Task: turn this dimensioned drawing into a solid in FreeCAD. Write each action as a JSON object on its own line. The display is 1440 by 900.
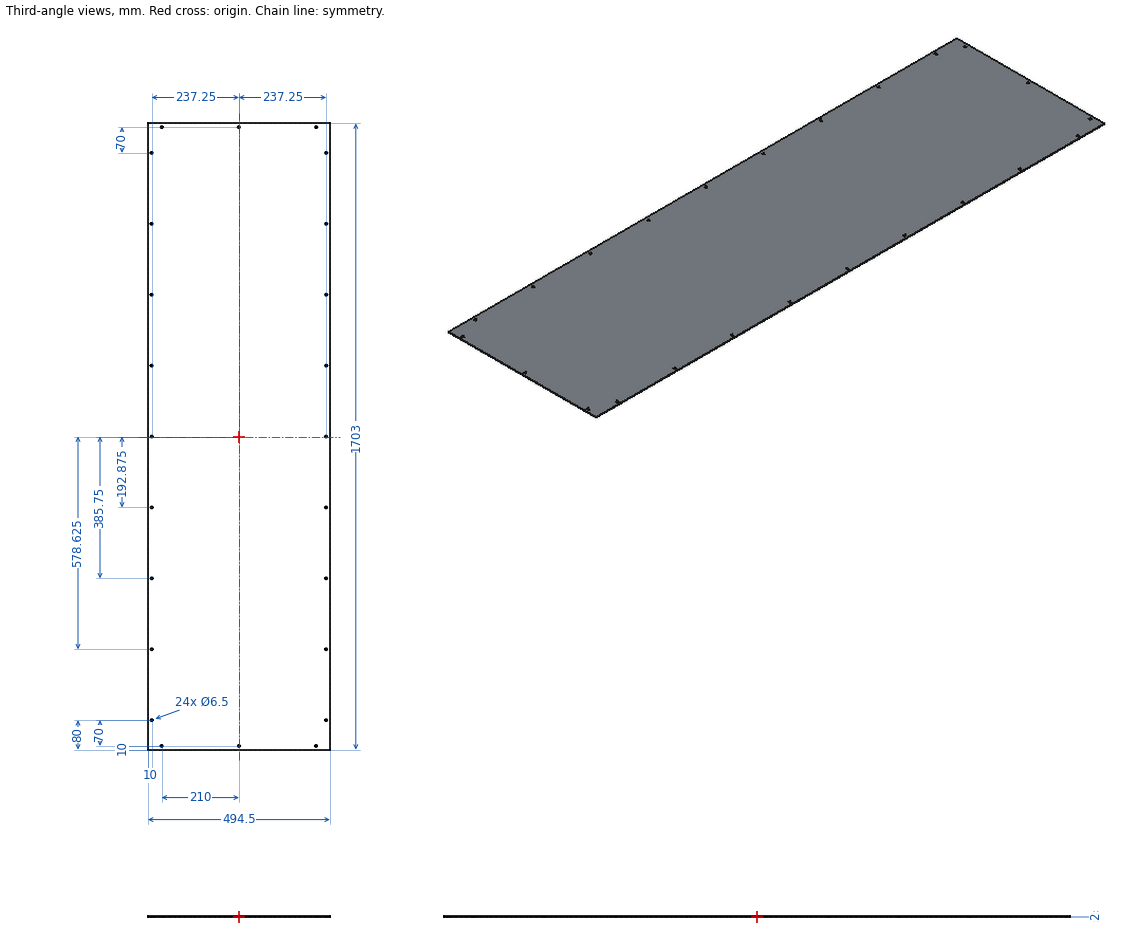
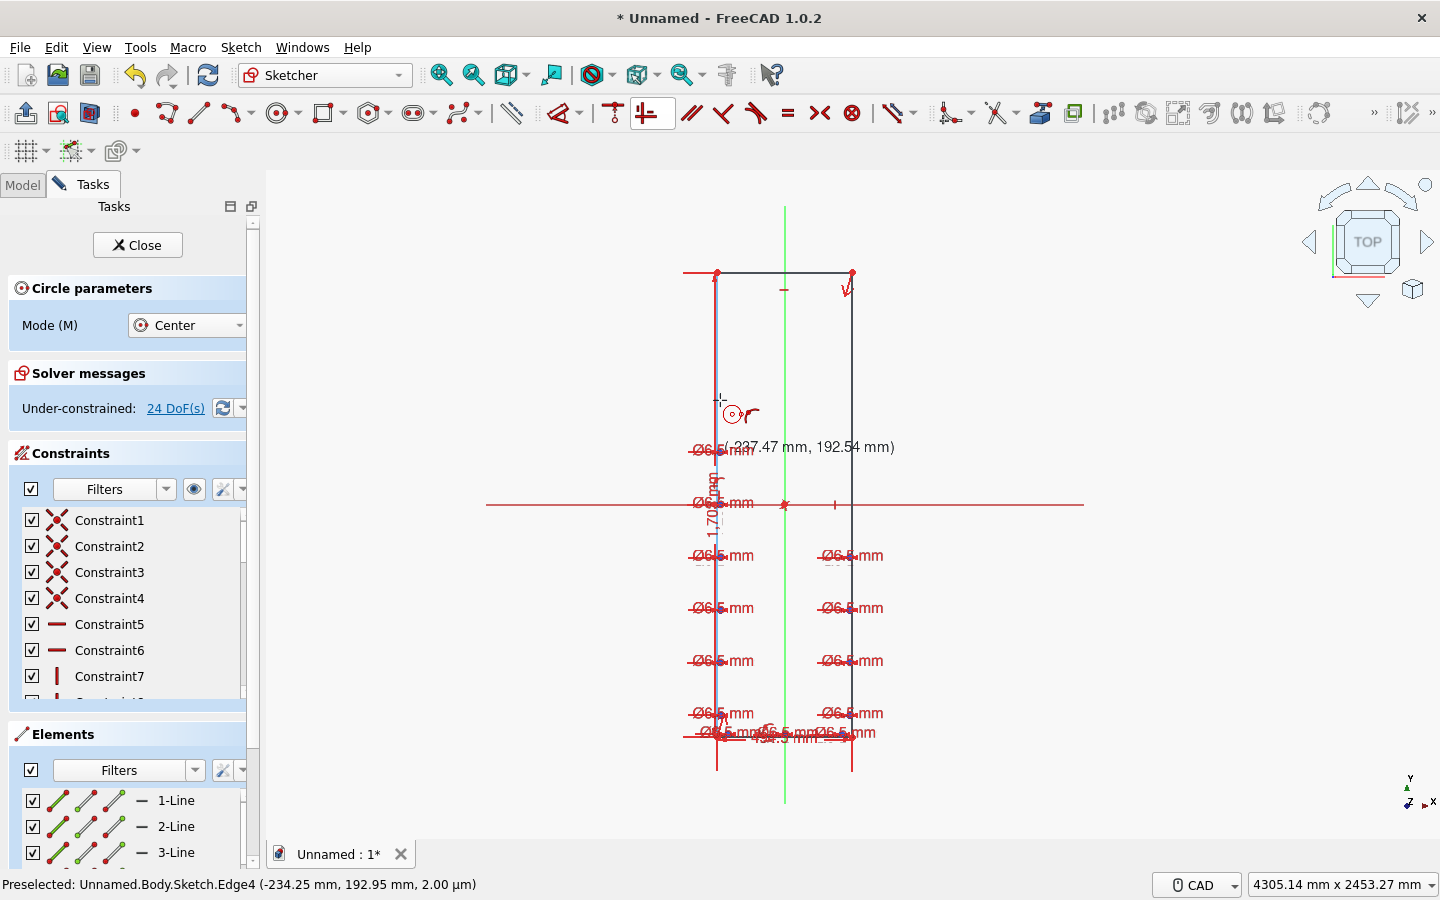
{"action": "scroll", "coordinate": [720, 400], "scroll_direction": "up", "scroll_amount": 9}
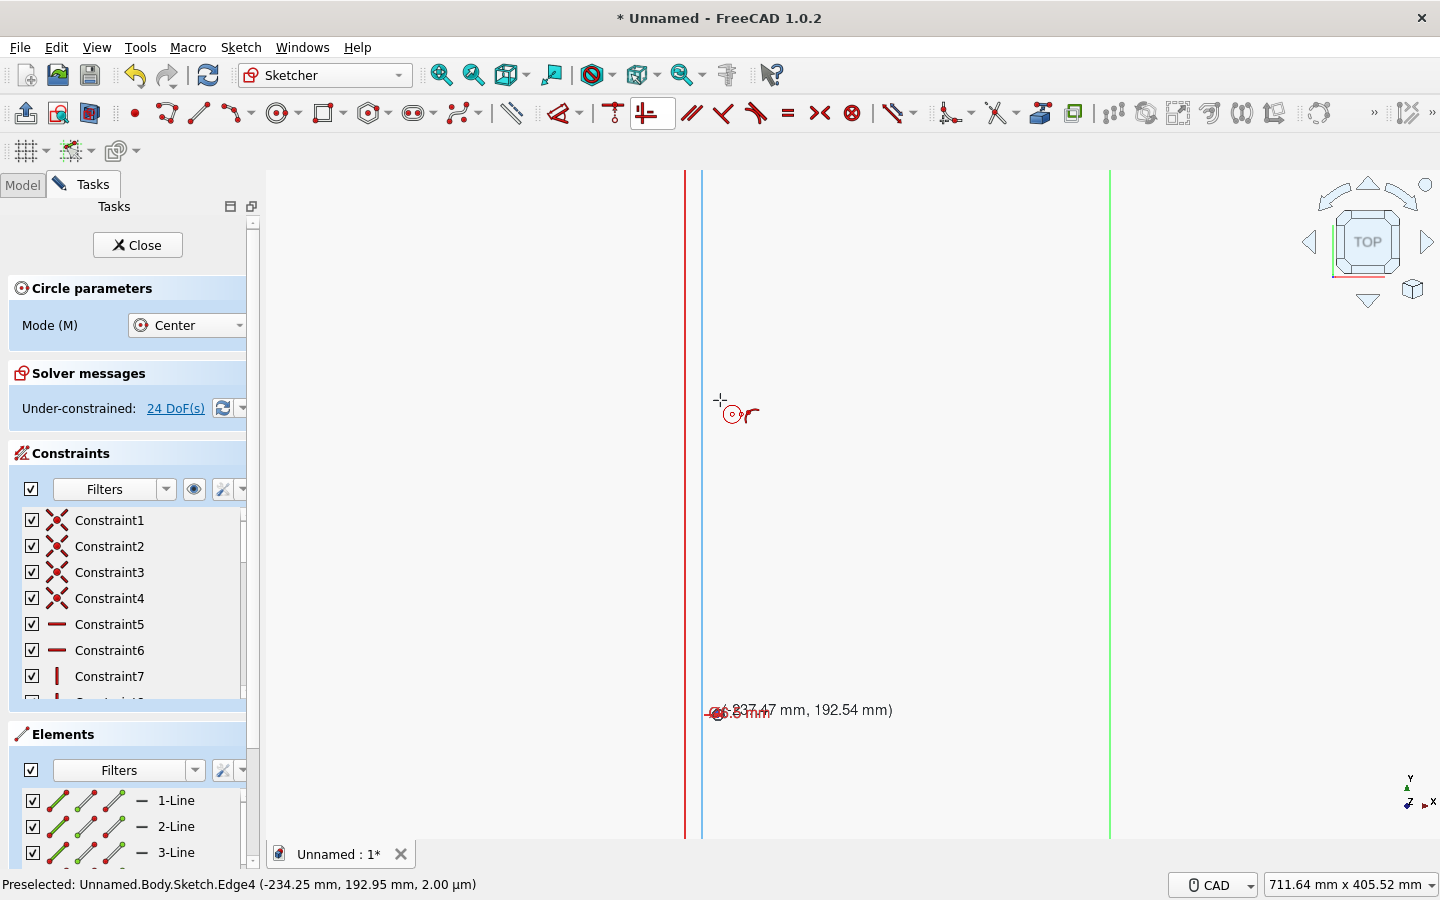
{"action": "left_click", "coordinate": [718, 396]}
{"action": "mouse_move", "coordinate": [722, 392]}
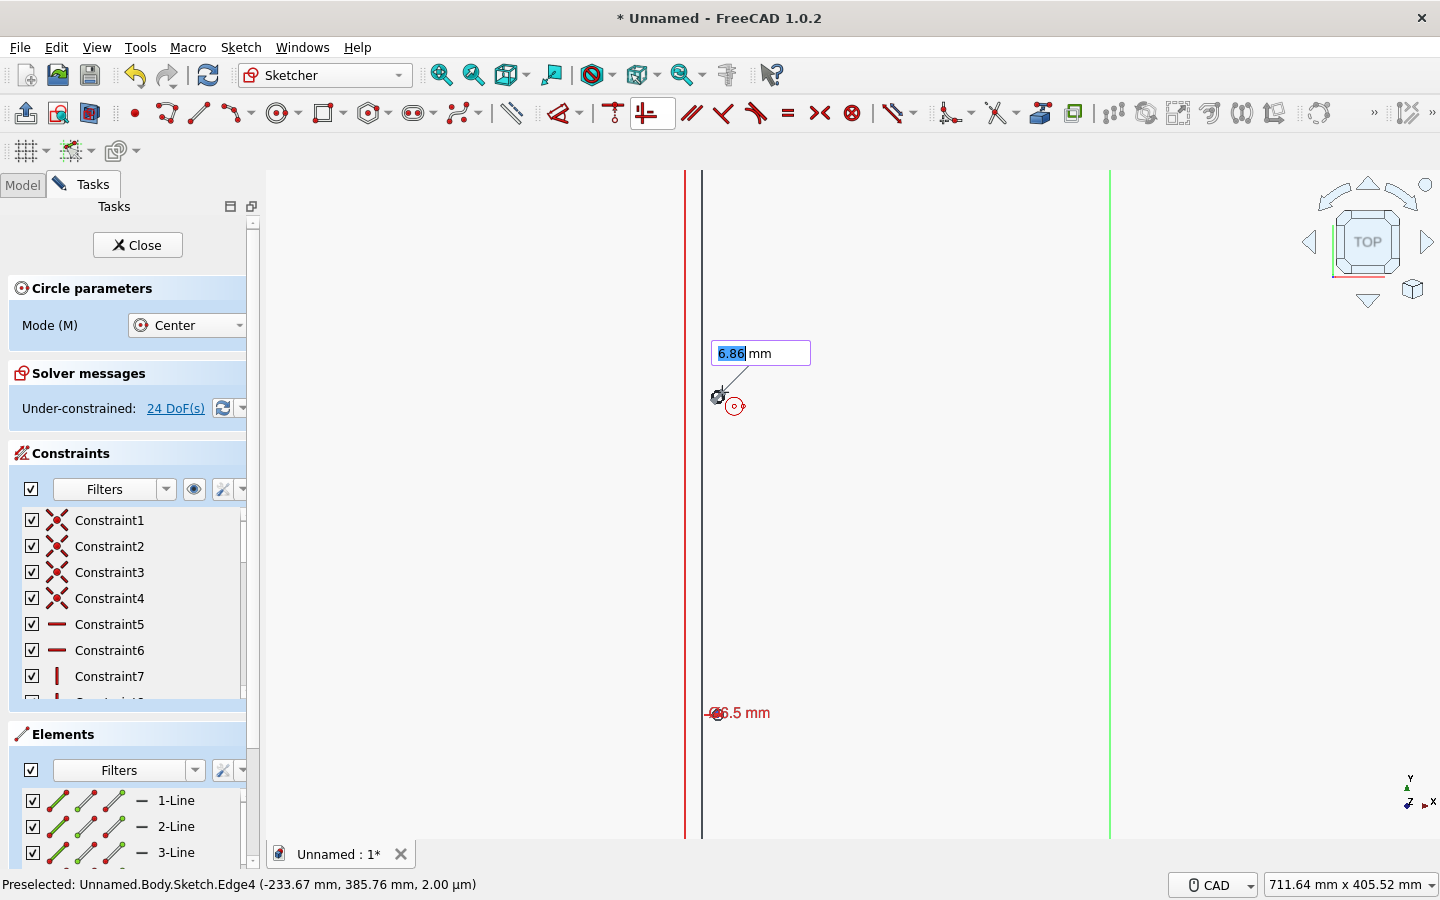
{"action": "type", "text": "6.5"}
{"action": "key", "text": "Return"}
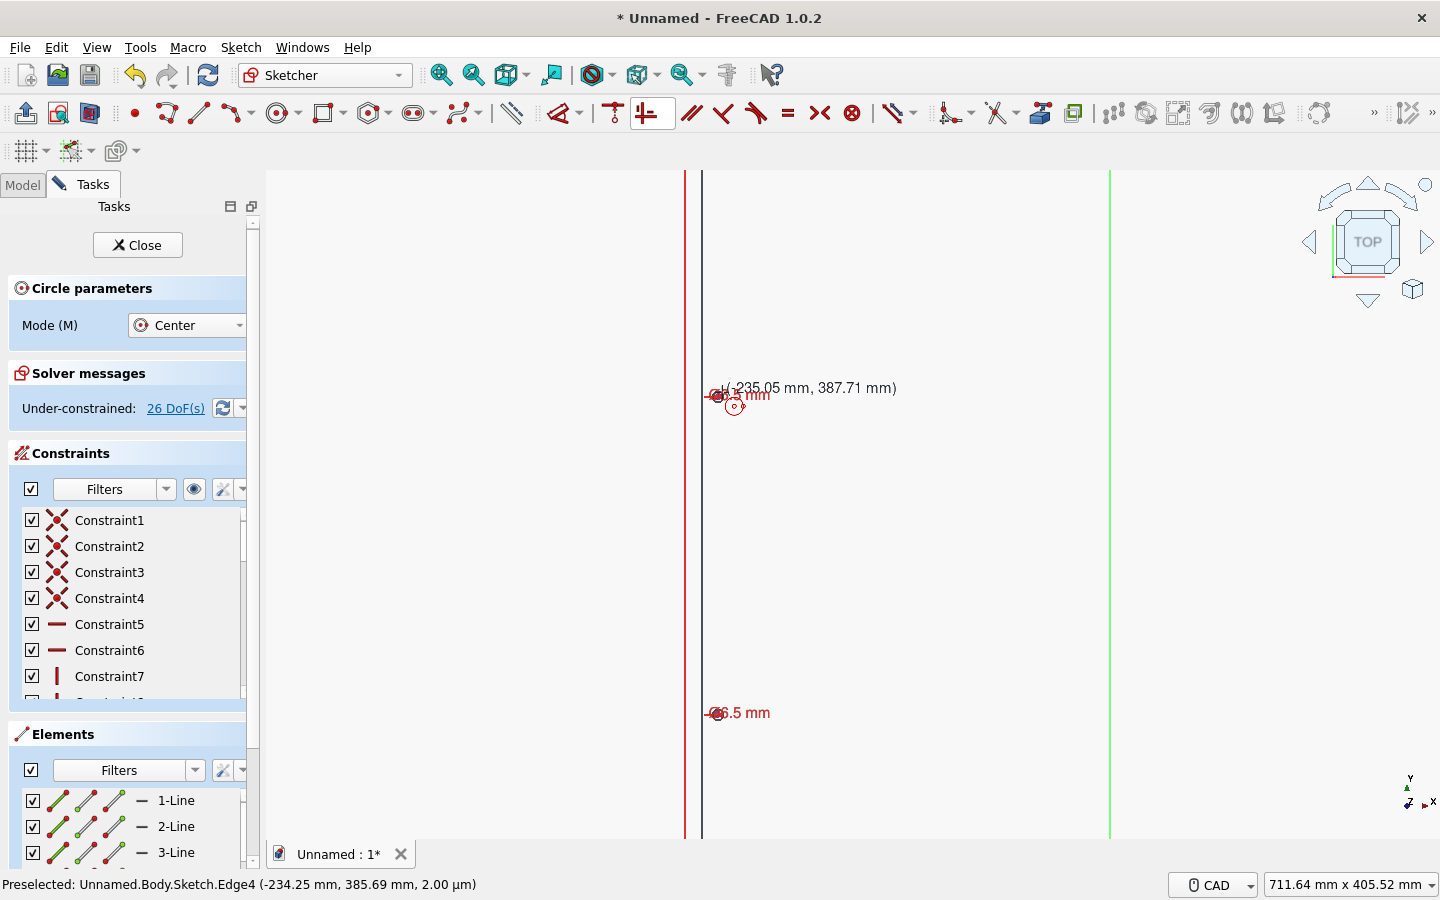
{"action": "scroll", "coordinate": [720, 400], "scroll_direction": "down", "scroll_amount": 9}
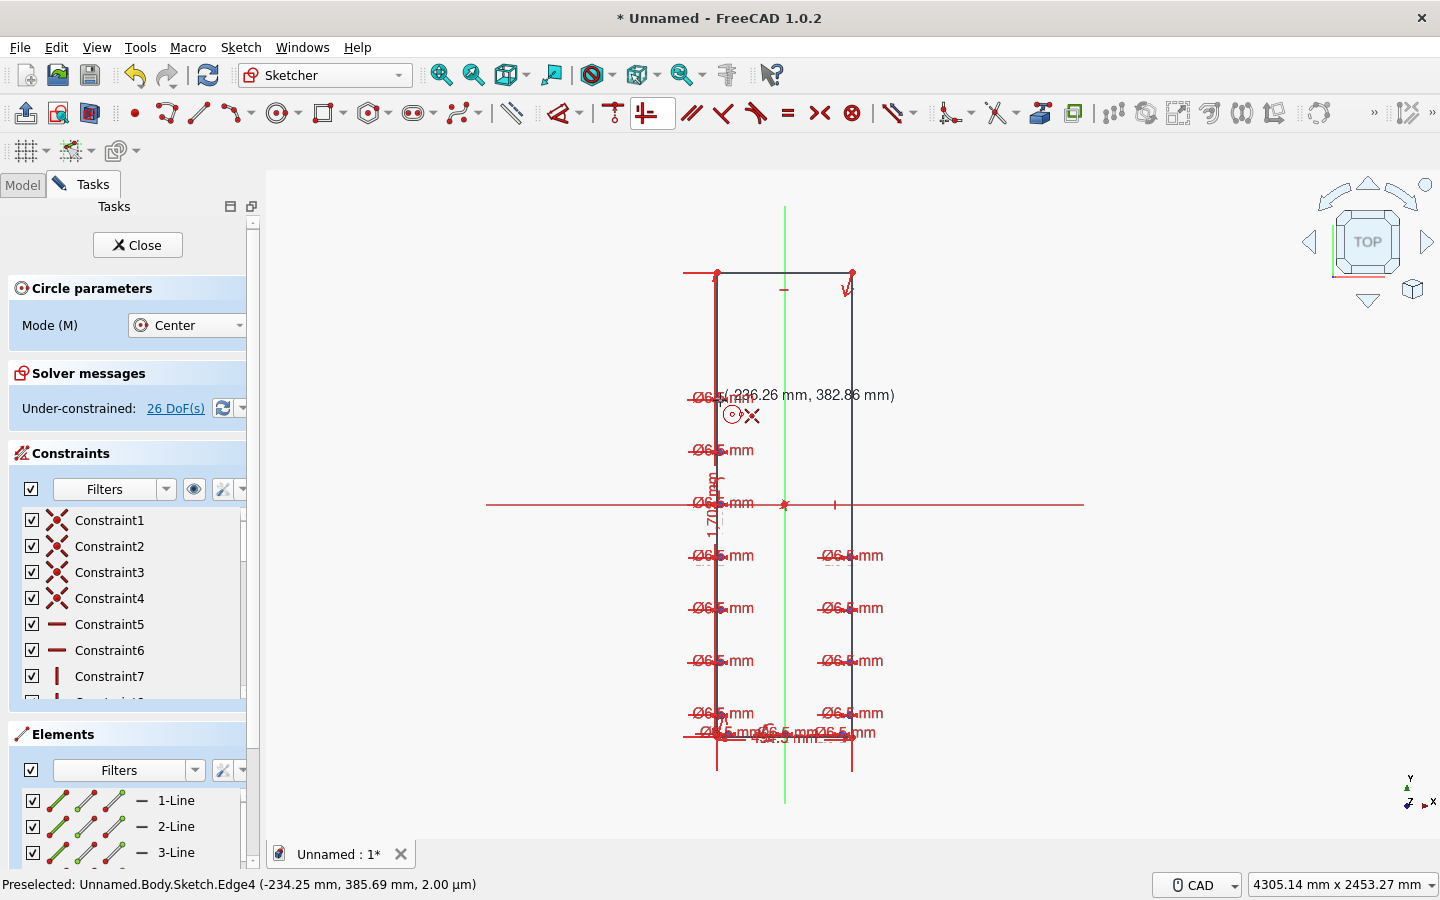
{"action": "scroll", "coordinate": [720, 347], "scroll_direction": "up", "scroll_amount": 17}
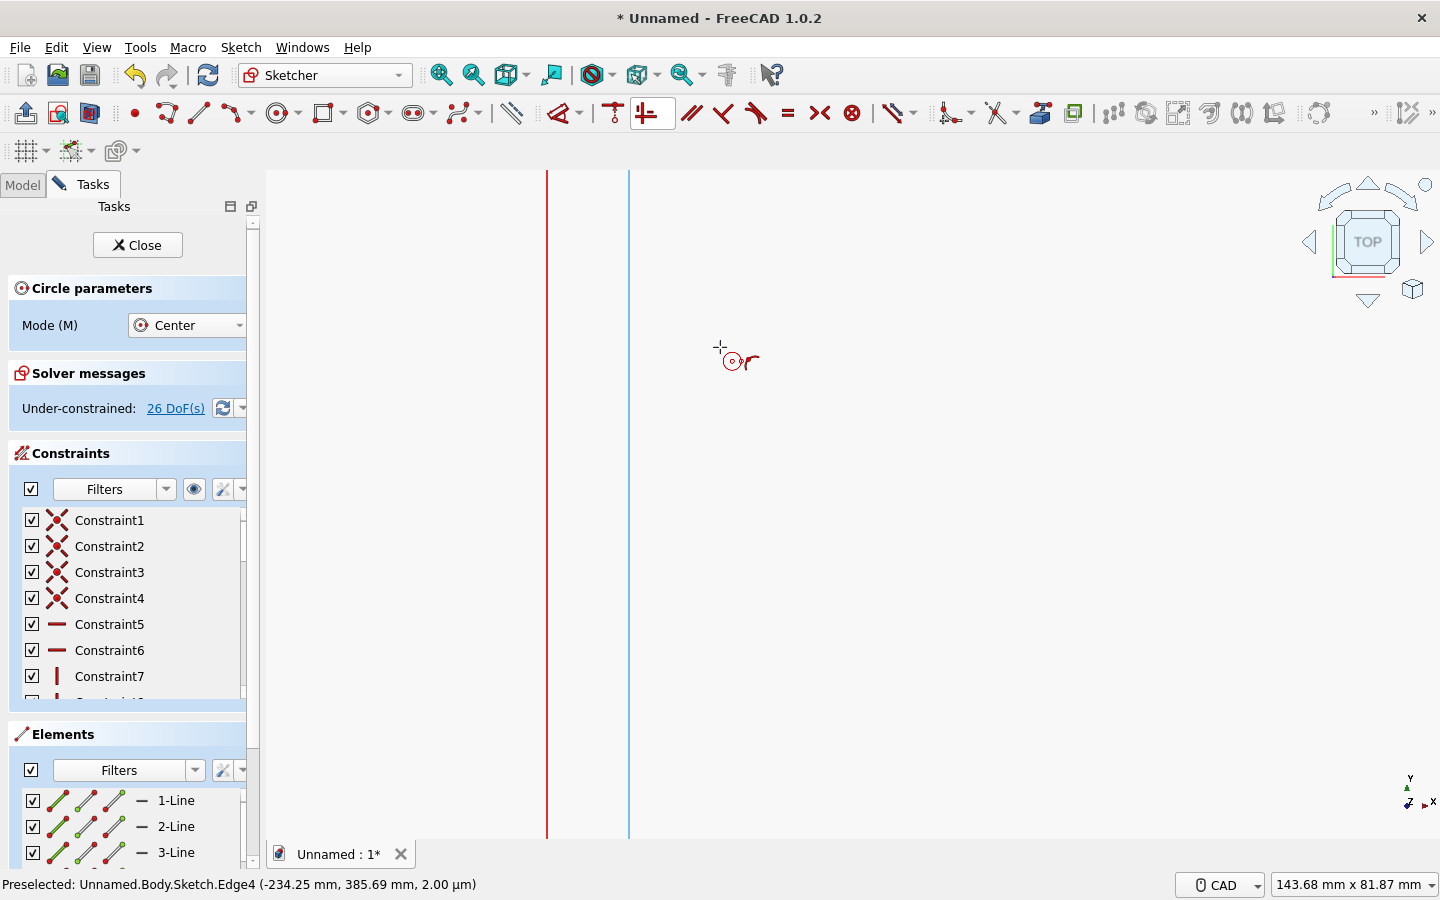
{"action": "scroll", "coordinate": [720, 347], "scroll_direction": "down", "scroll_amount": 17}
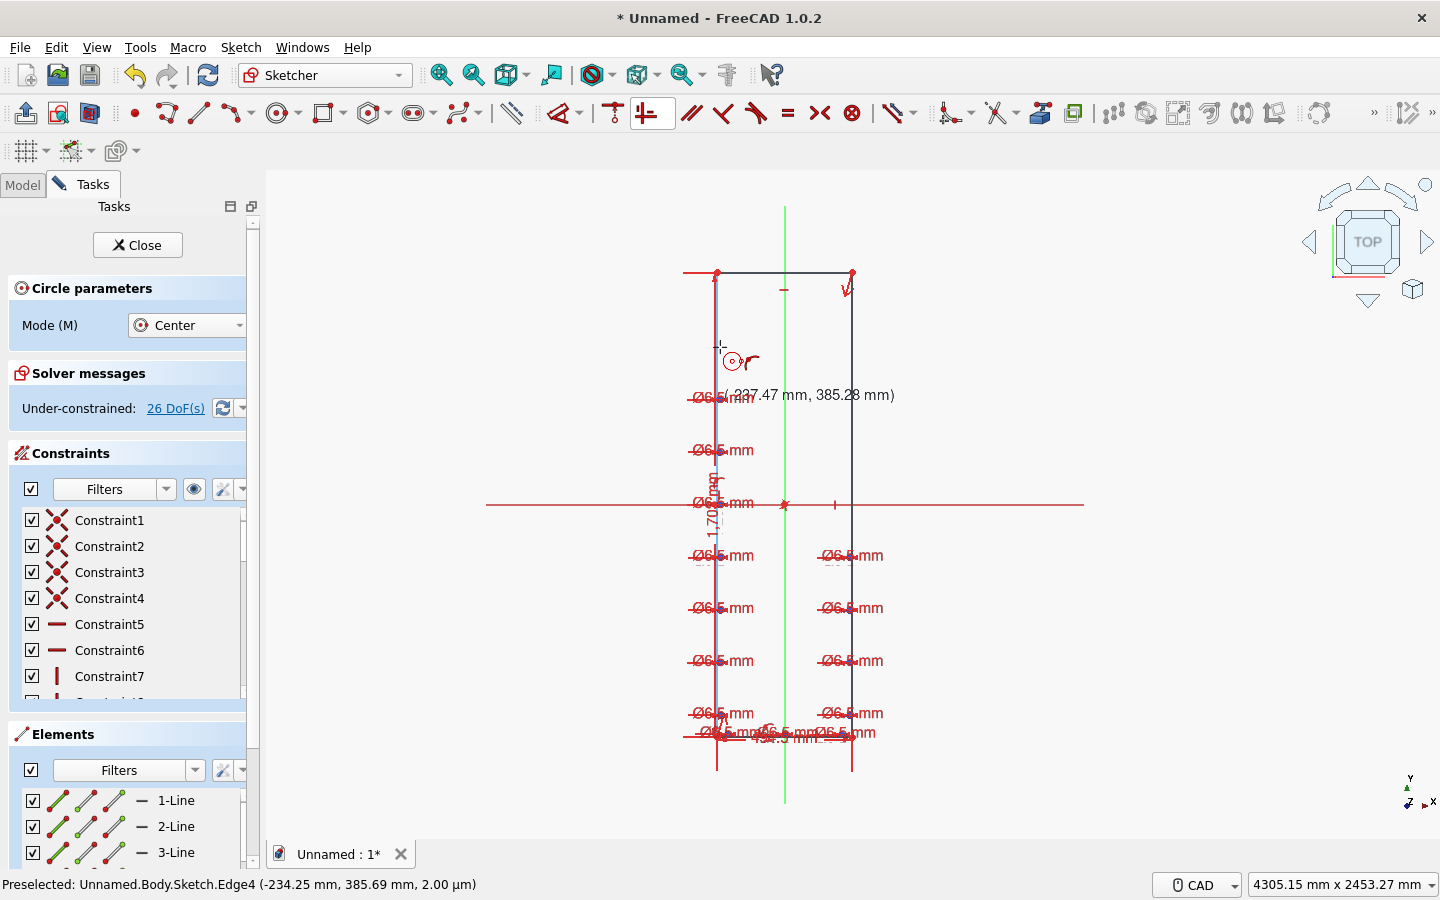
{"action": "scroll", "coordinate": [720, 347], "scroll_direction": "up", "scroll_amount": 9}